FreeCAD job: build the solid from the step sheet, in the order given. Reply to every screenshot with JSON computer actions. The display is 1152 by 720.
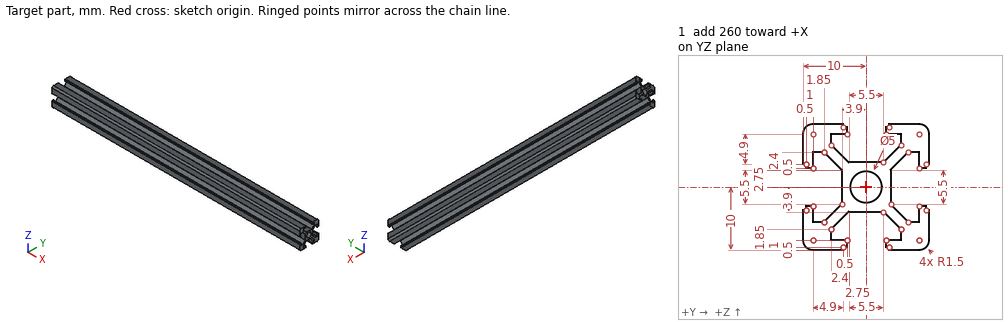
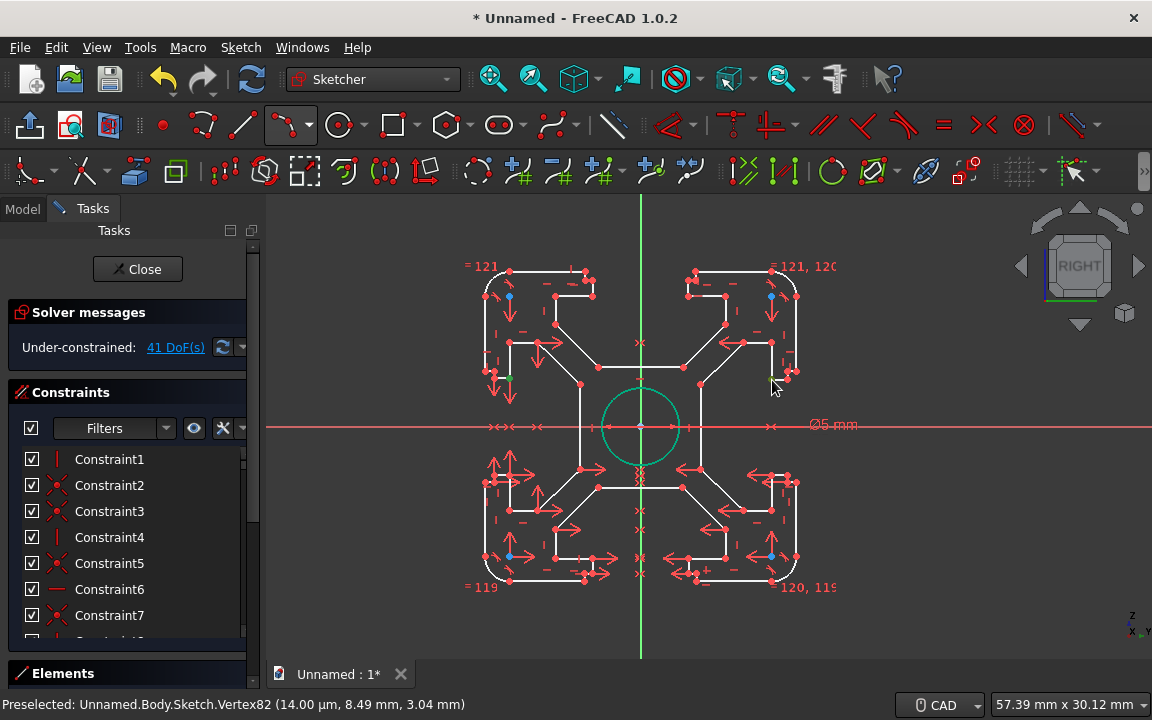
{"action": "left_click", "coordinate": [641, 602]}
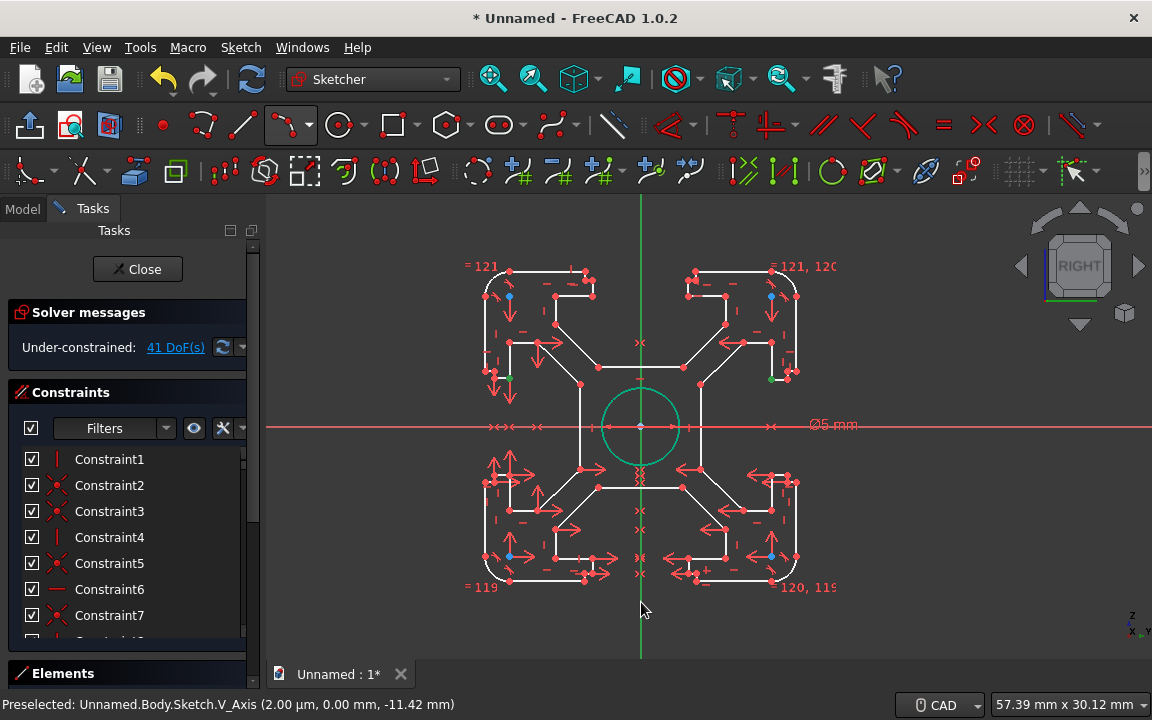
{"action": "key", "text": "s"}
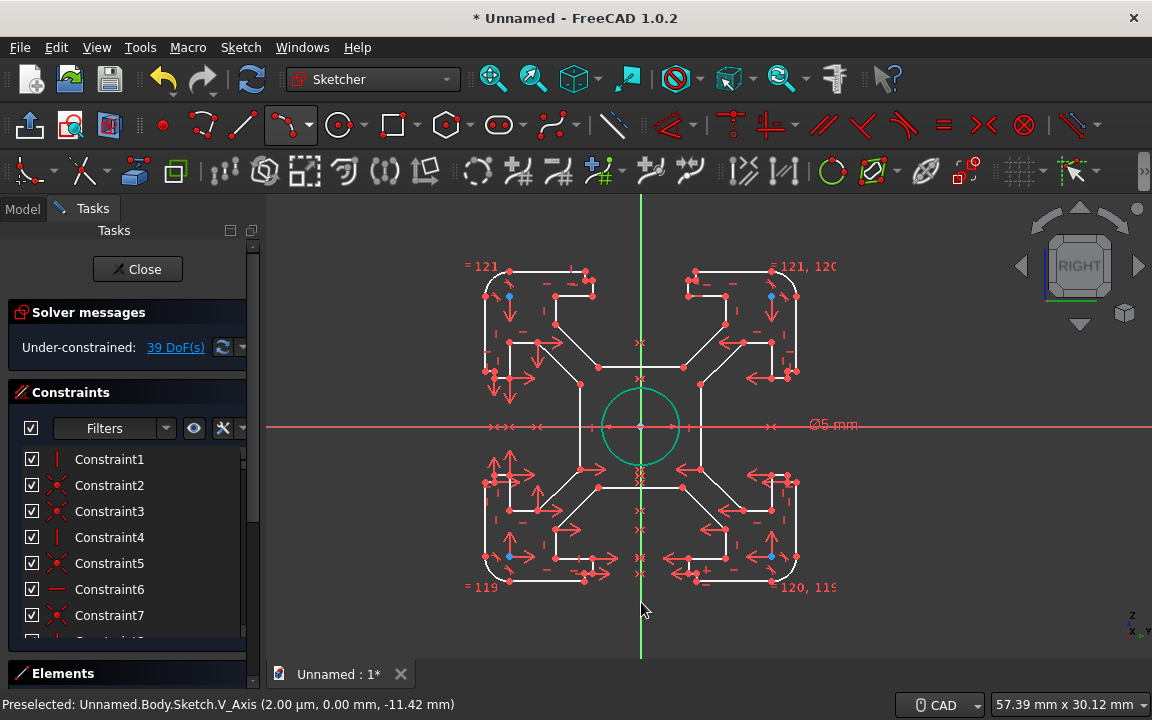
{"action": "scroll", "coordinate": [494, 371], "scroll_direction": "up", "scroll_amount": 3}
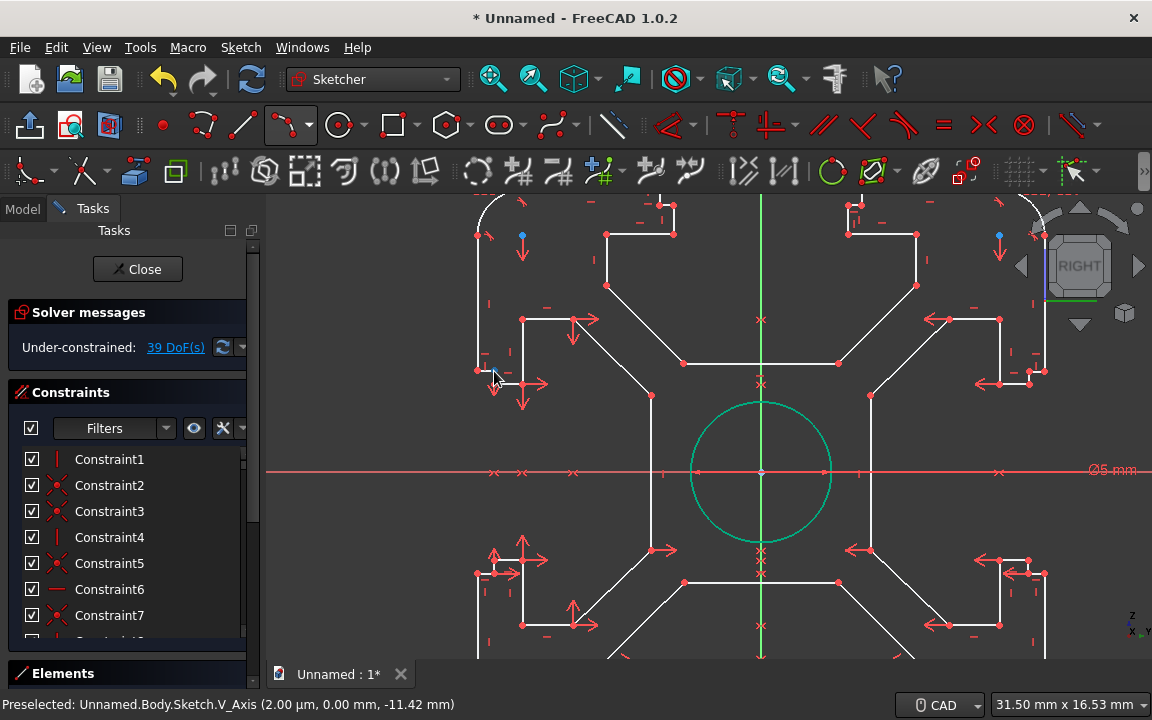
{"action": "left_click", "coordinate": [494, 371]}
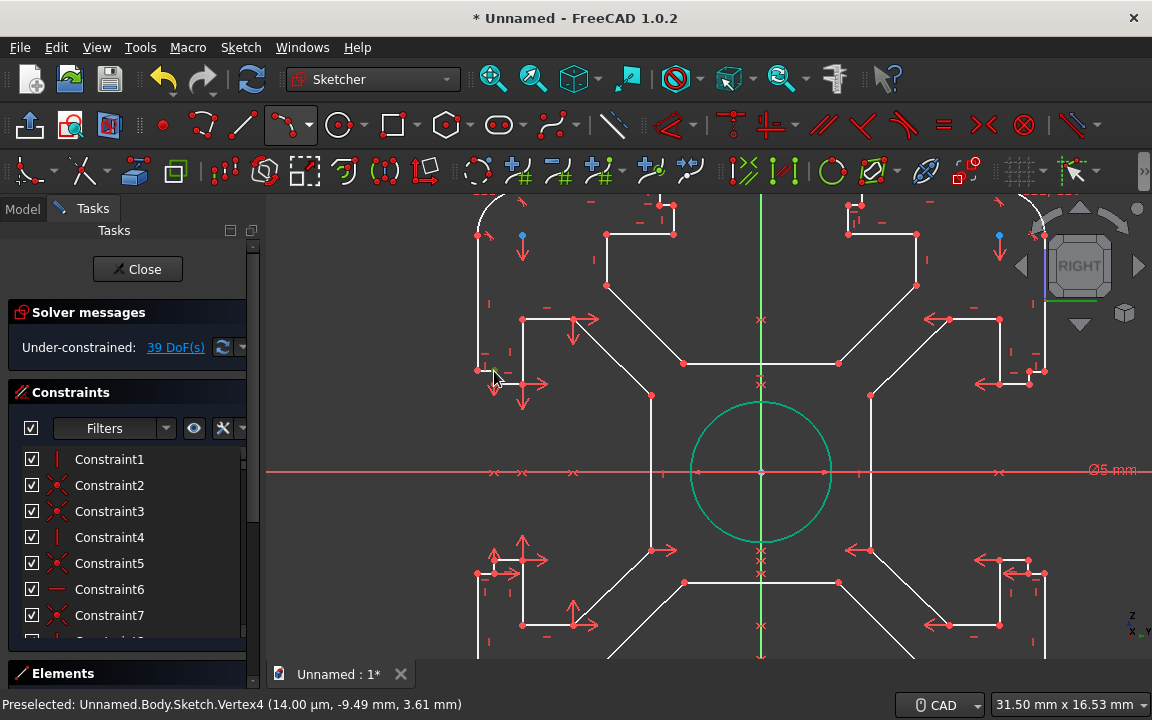
{"action": "scroll", "coordinate": [494, 371], "scroll_direction": "down", "scroll_amount": 3}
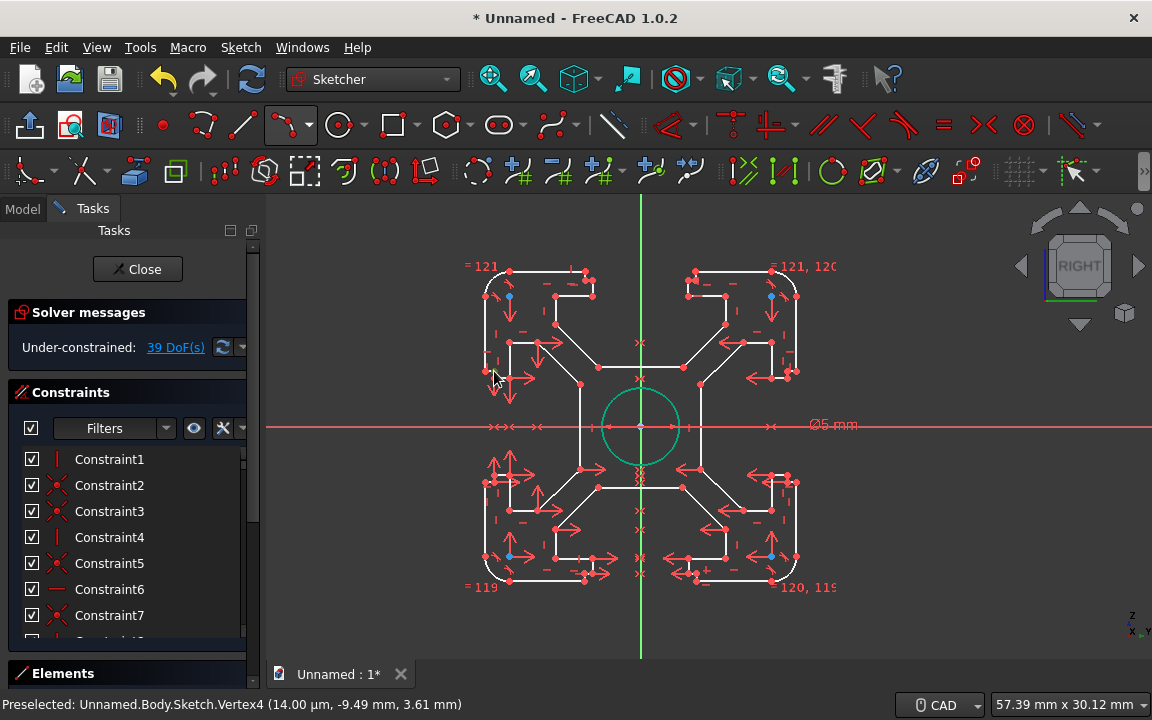
{"action": "scroll", "coordinate": [788, 371], "scroll_direction": "up", "scroll_amount": 3}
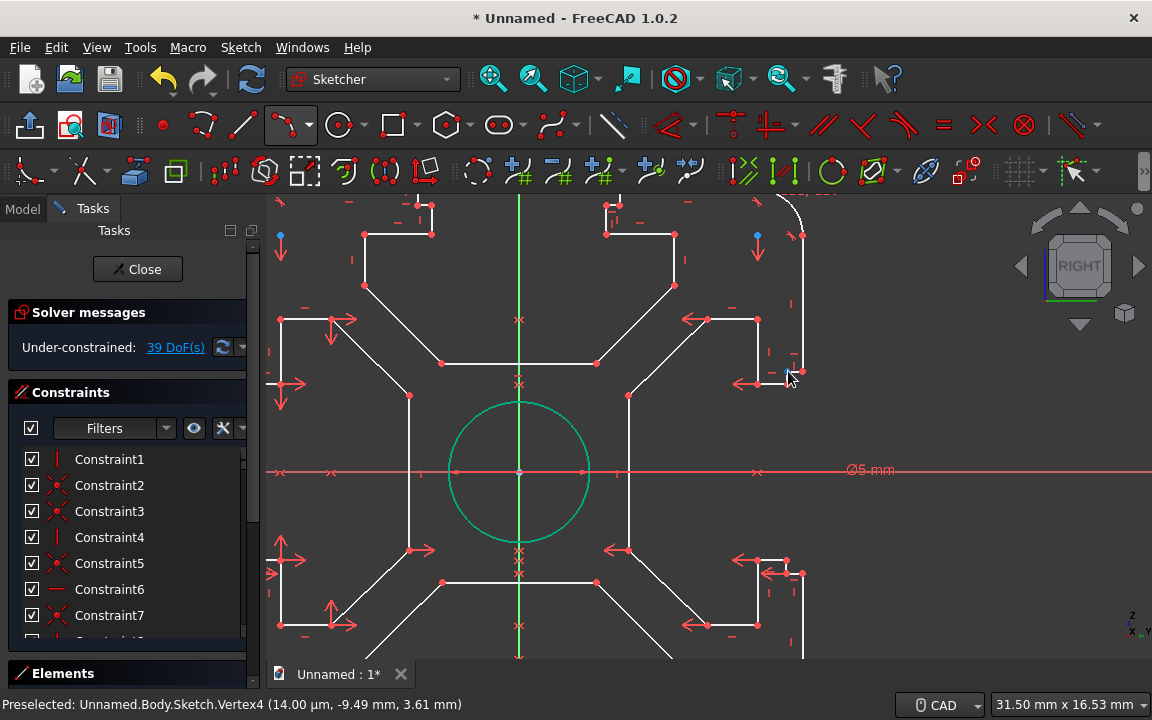
{"action": "left_click", "coordinate": [787, 372]}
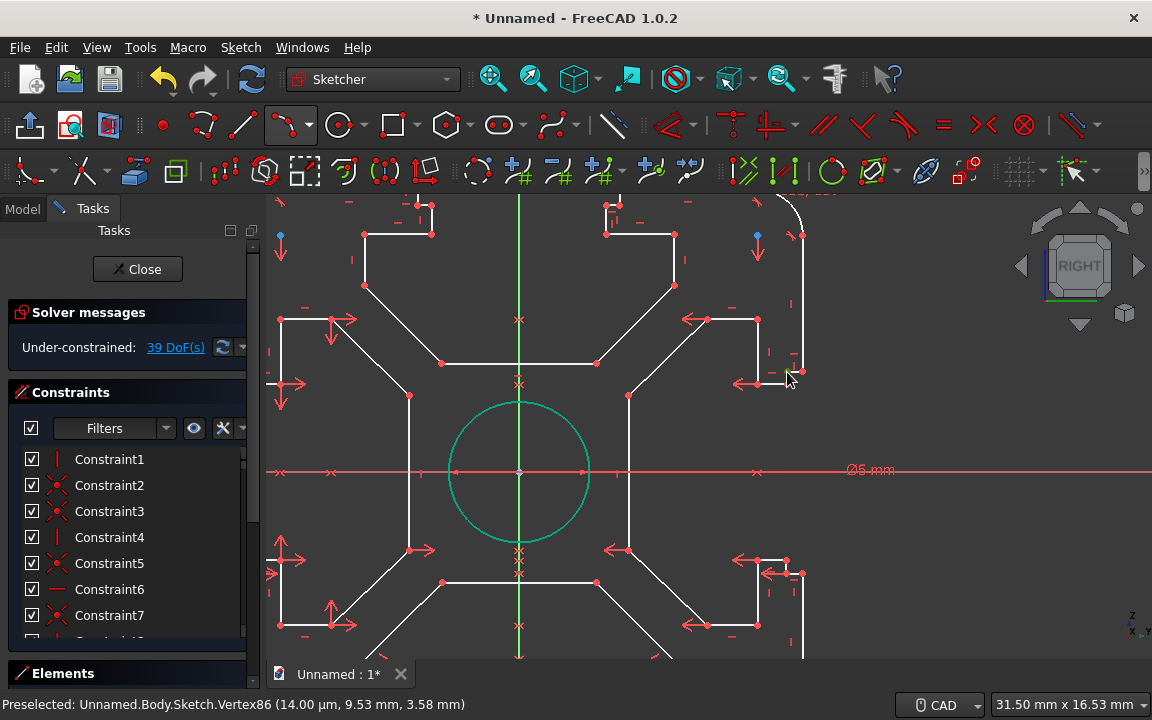
{"action": "left_click", "coordinate": [519, 310]}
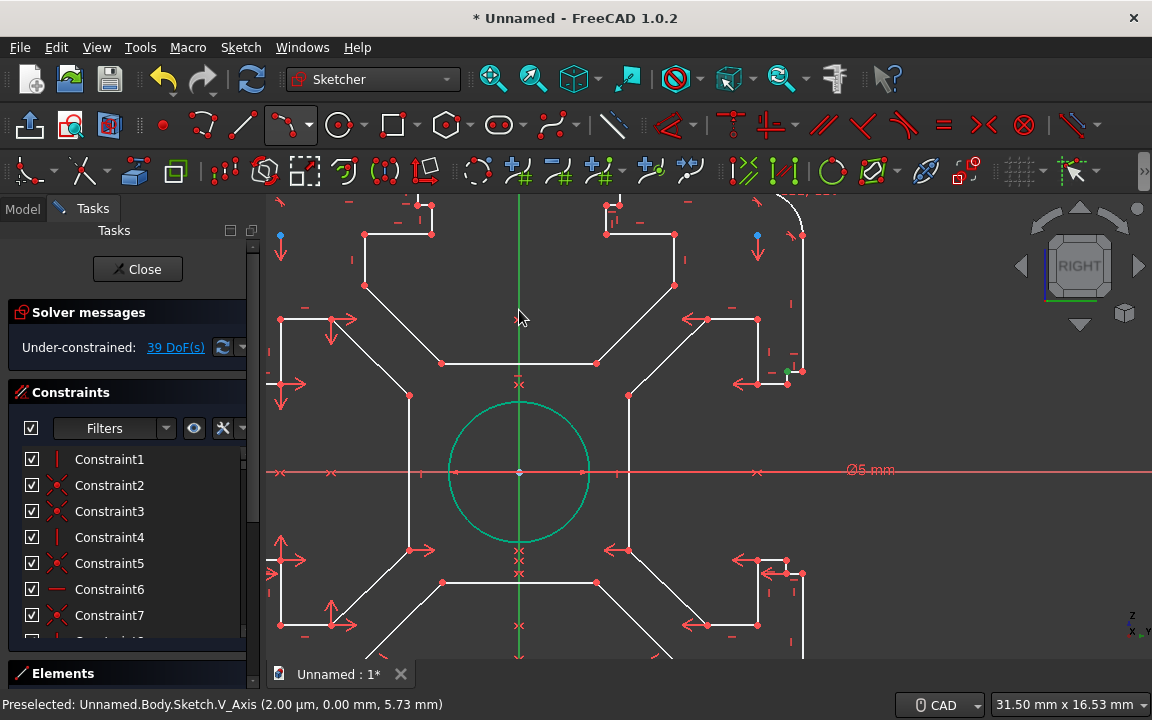
{"action": "key", "text": "s"}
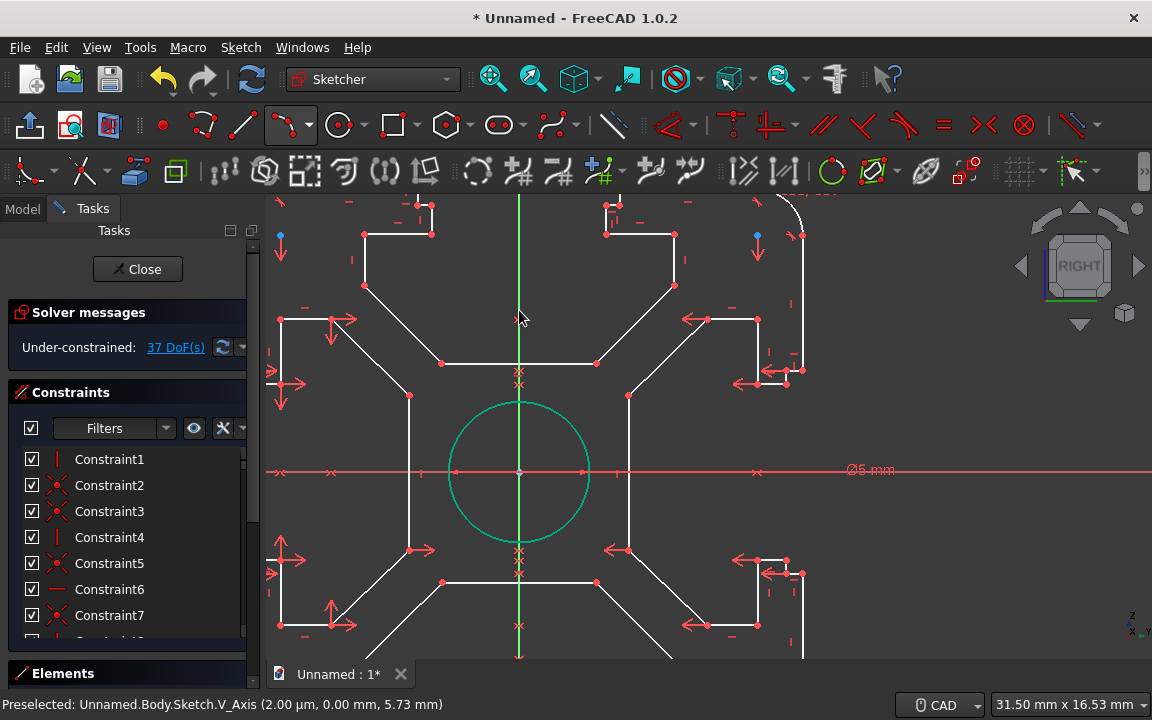
{"action": "scroll", "coordinate": [788, 371], "scroll_direction": "down", "scroll_amount": 3}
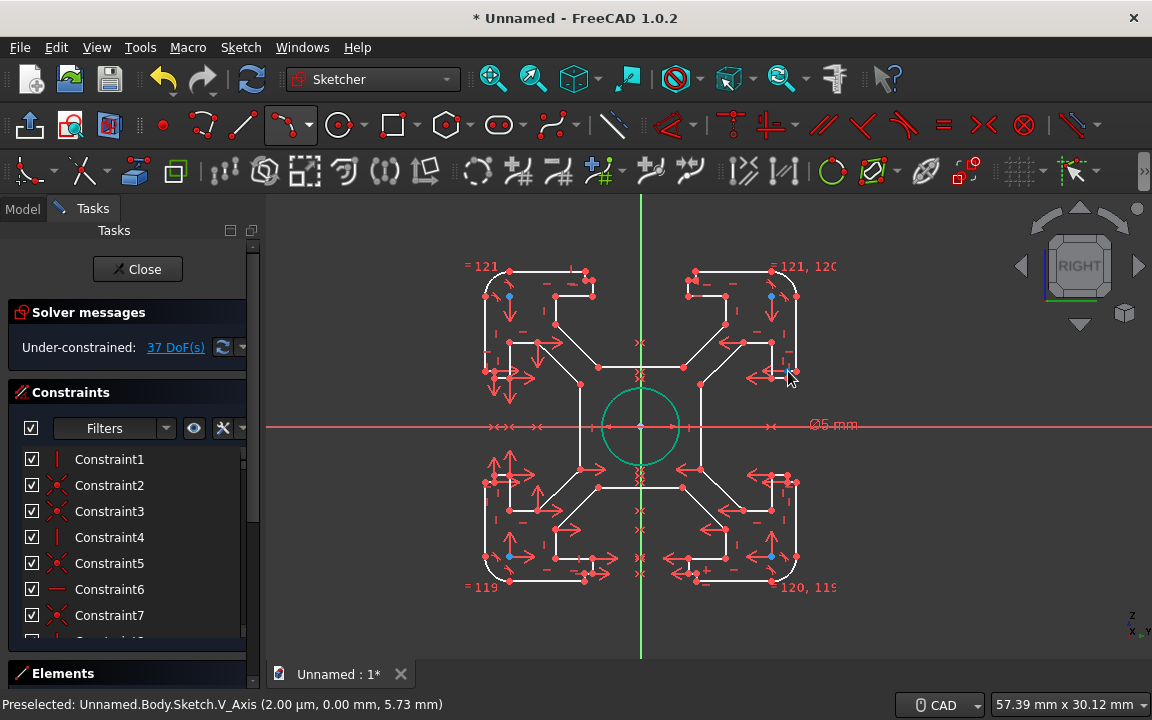
{"action": "scroll", "coordinate": [697, 574], "scroll_direction": "up", "scroll_amount": 3}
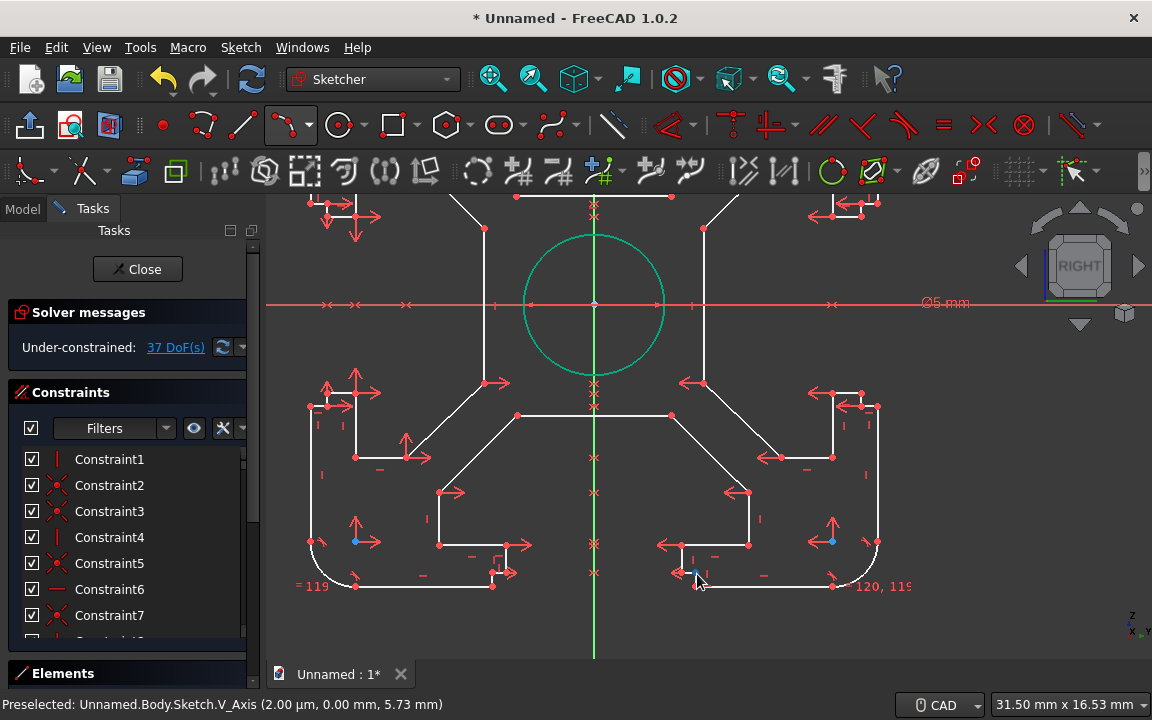
{"action": "left_click", "coordinate": [696, 573]}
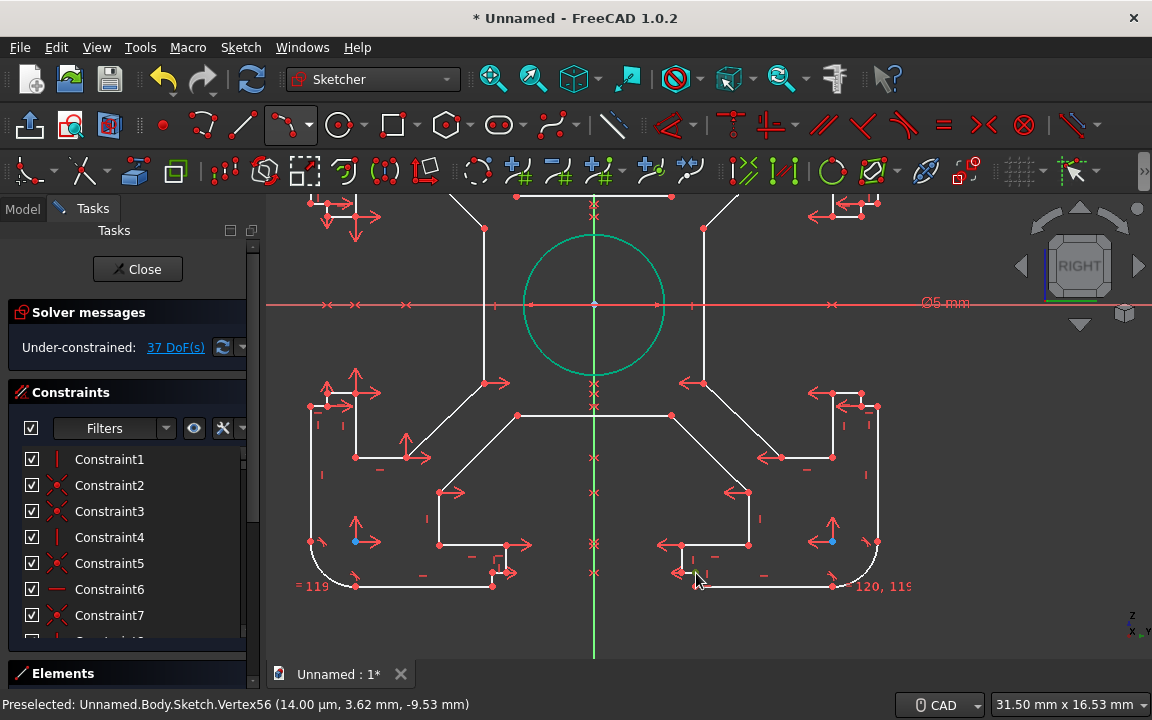
{"action": "scroll", "coordinate": [697, 574], "scroll_direction": "down", "scroll_amount": 3}